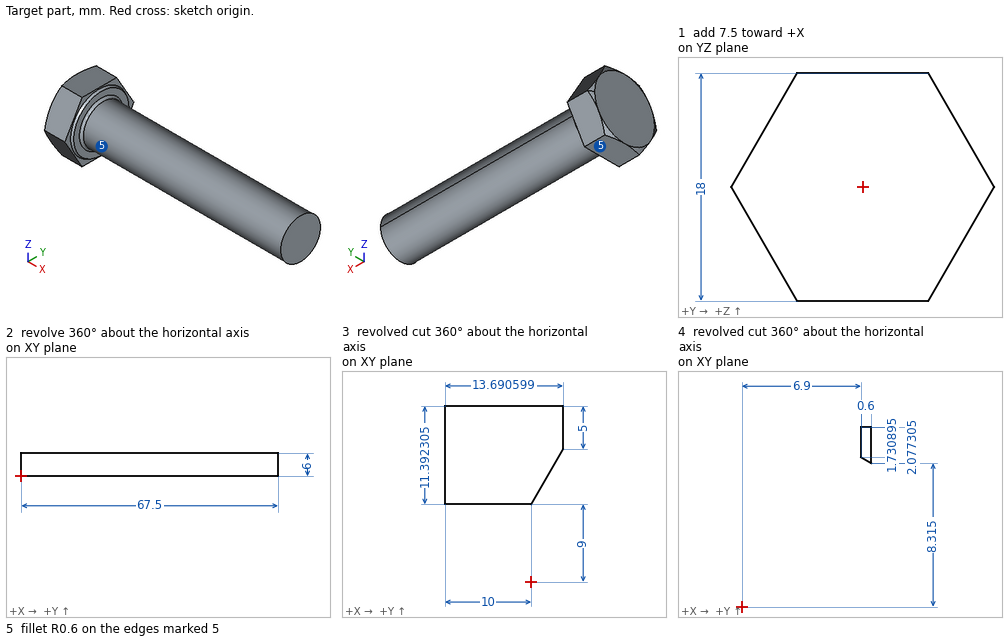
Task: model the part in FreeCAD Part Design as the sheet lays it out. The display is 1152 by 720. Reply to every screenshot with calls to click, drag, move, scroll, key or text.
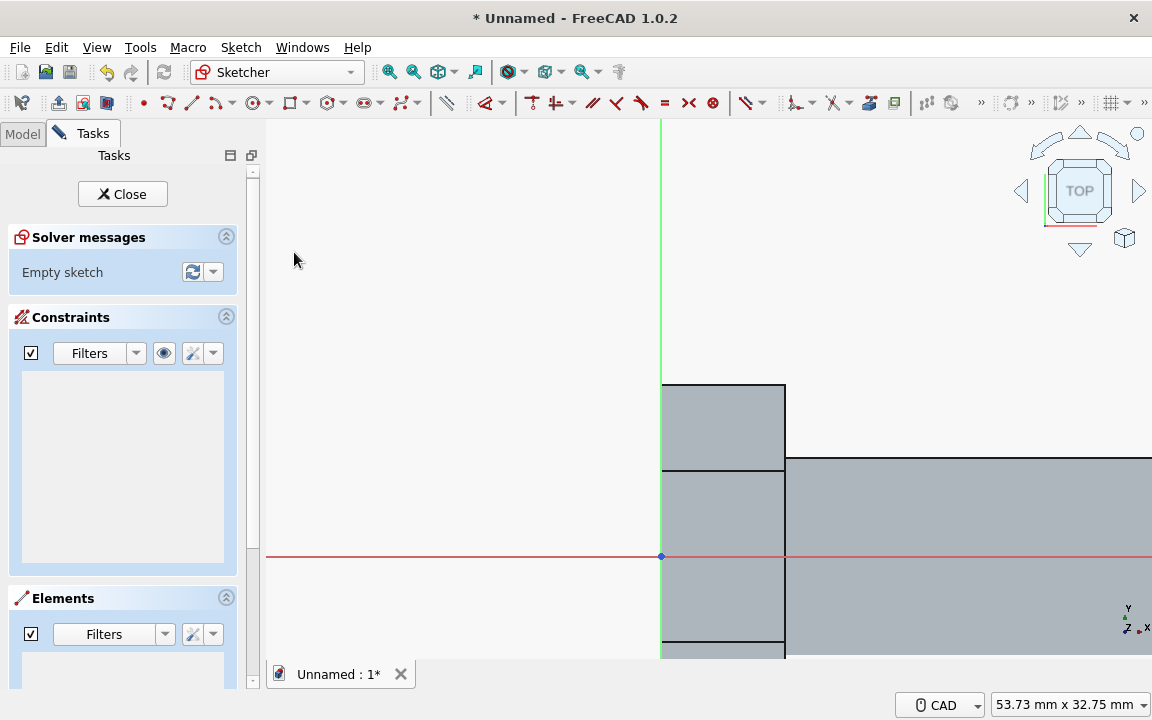
click(168, 104)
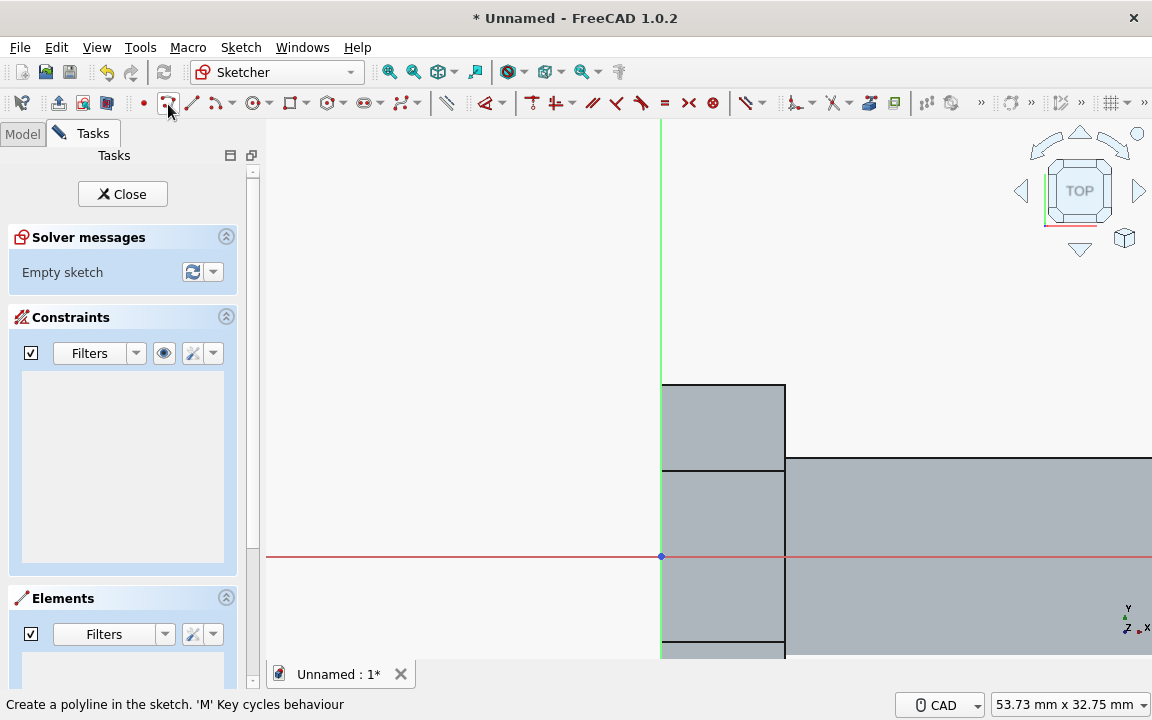
click(661, 408)
click(722, 303)
click(722, 220)
click(496, 220)
click(496, 408)
click(661, 409)
key(Escape)
key(Escape)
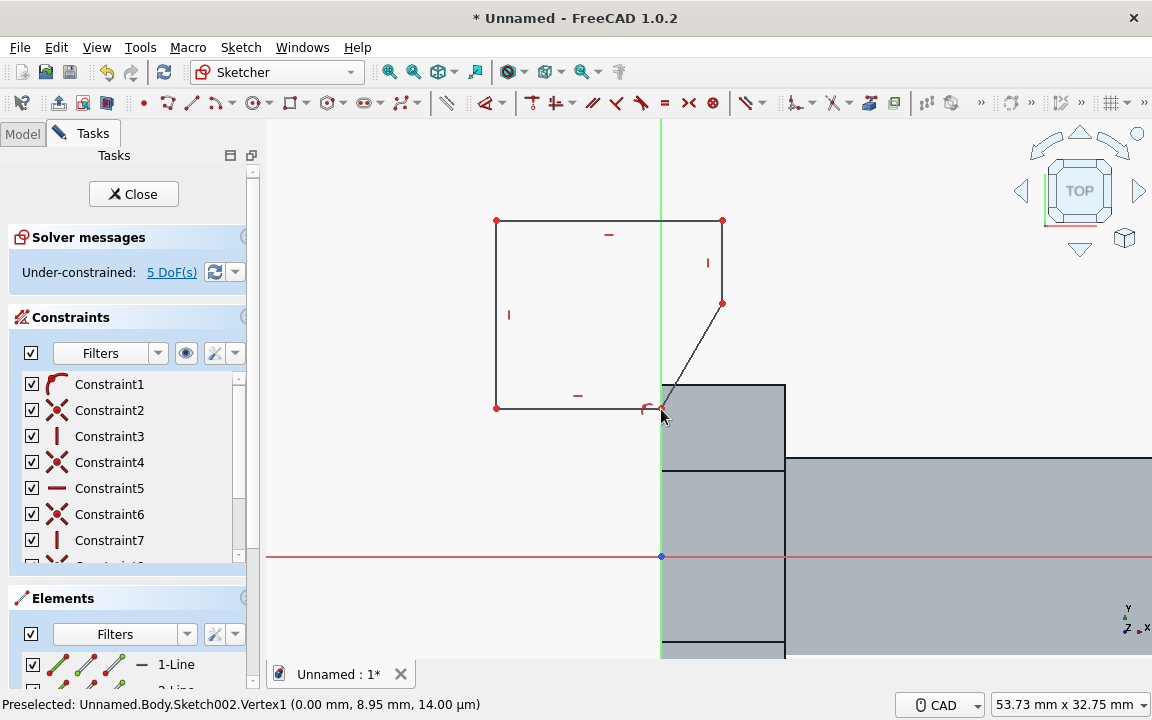
click(486, 104)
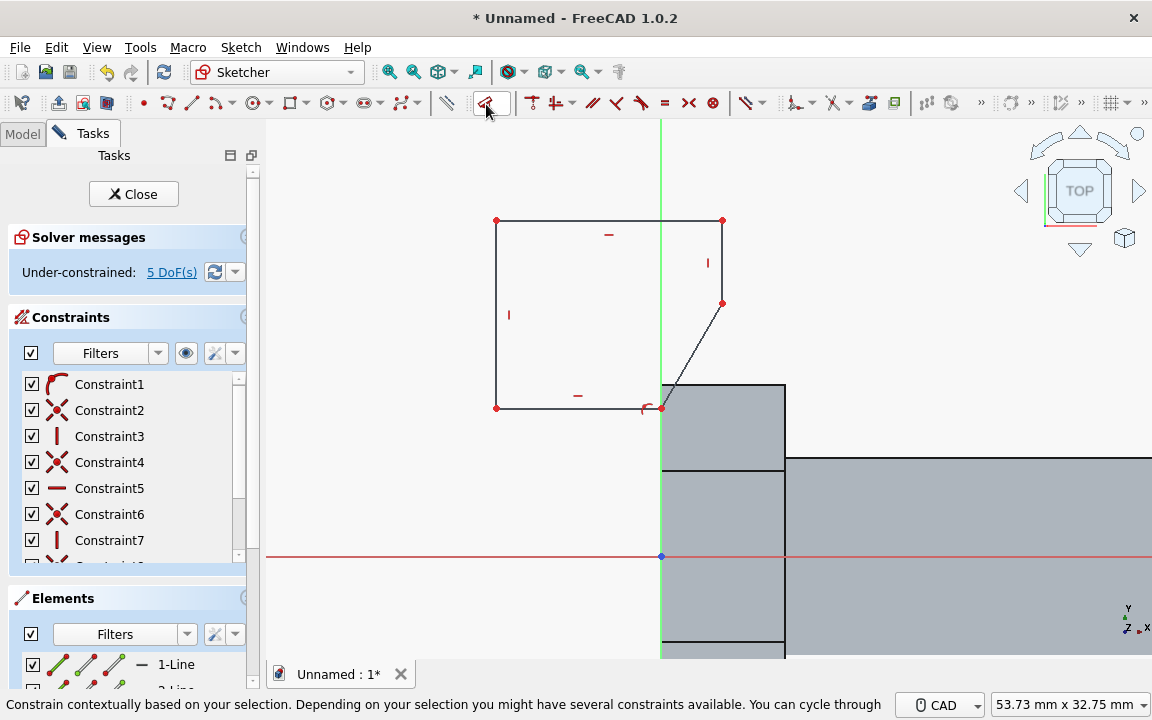
click(722, 279)
click(756, 262)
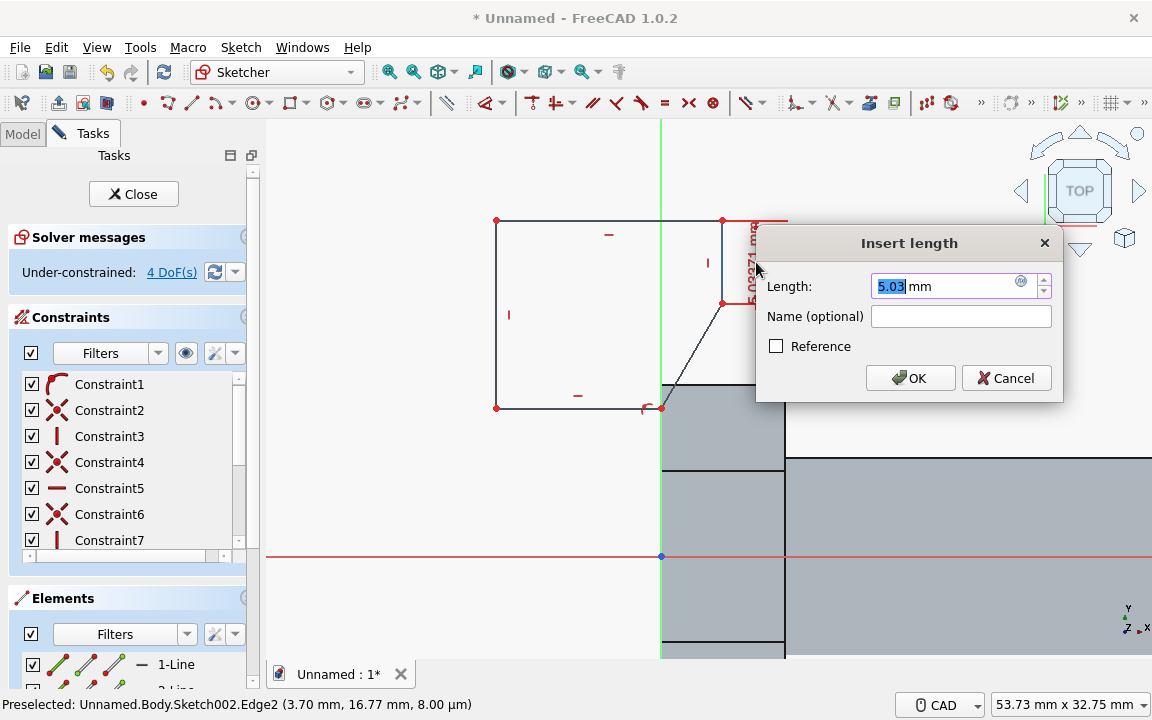
text(5)
key(Return)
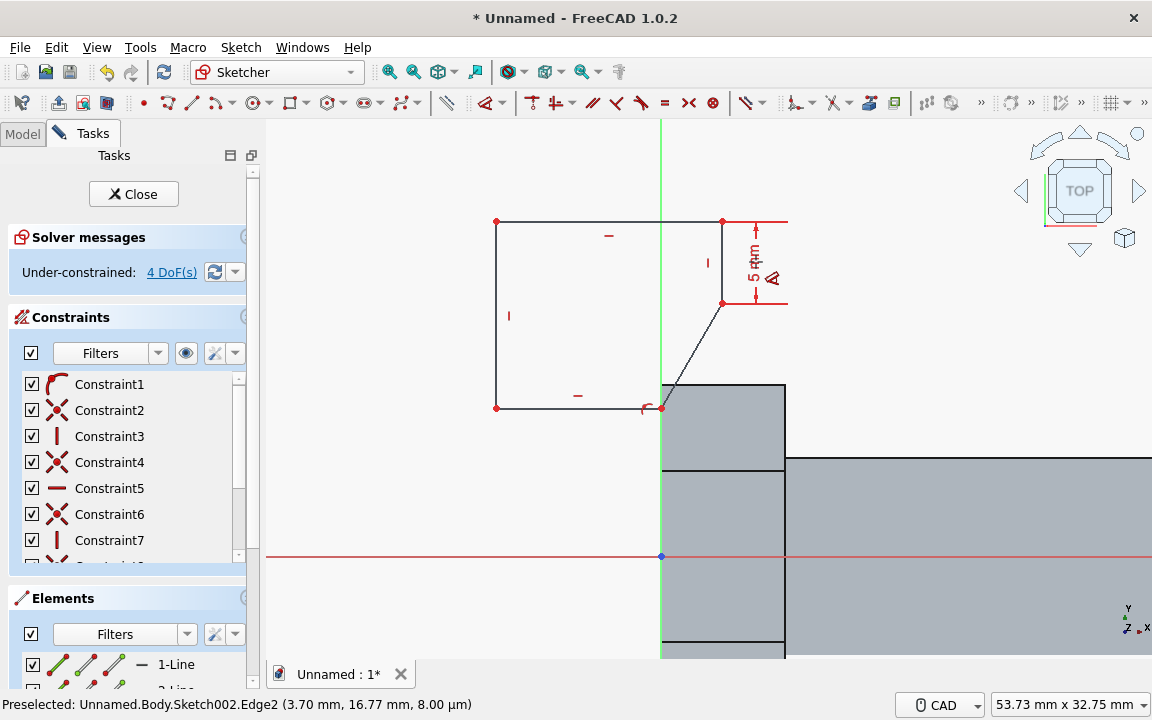
click(546, 409)
click(579, 443)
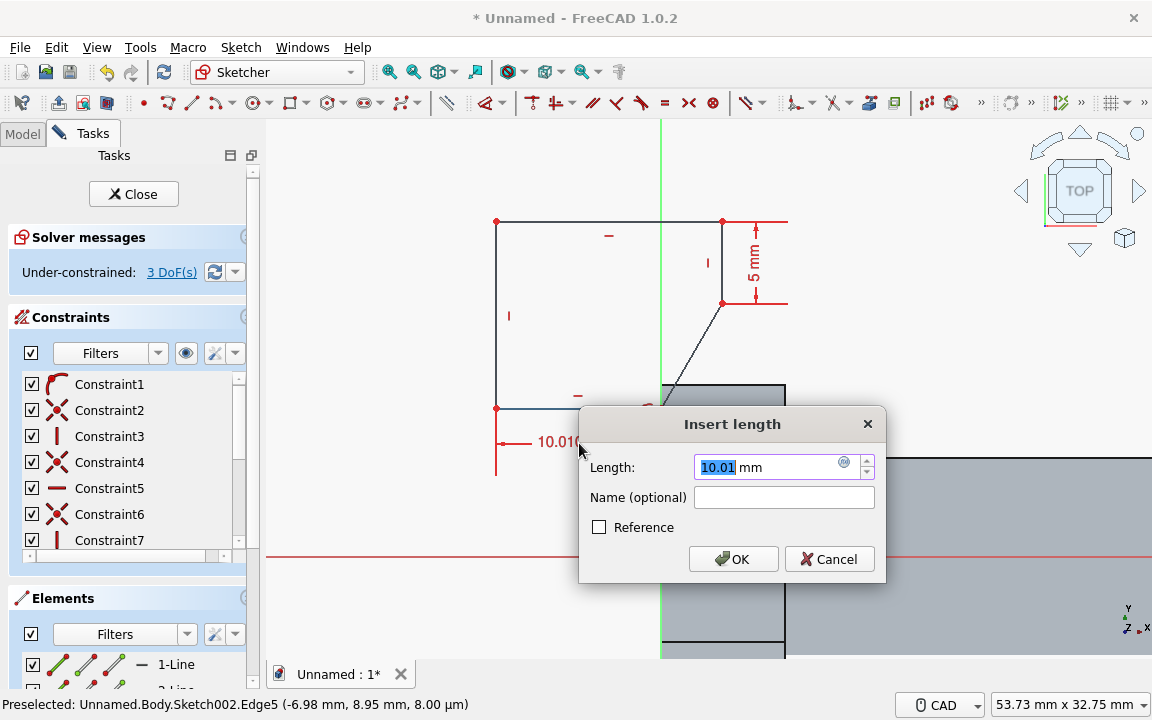
text(10)
key(Return)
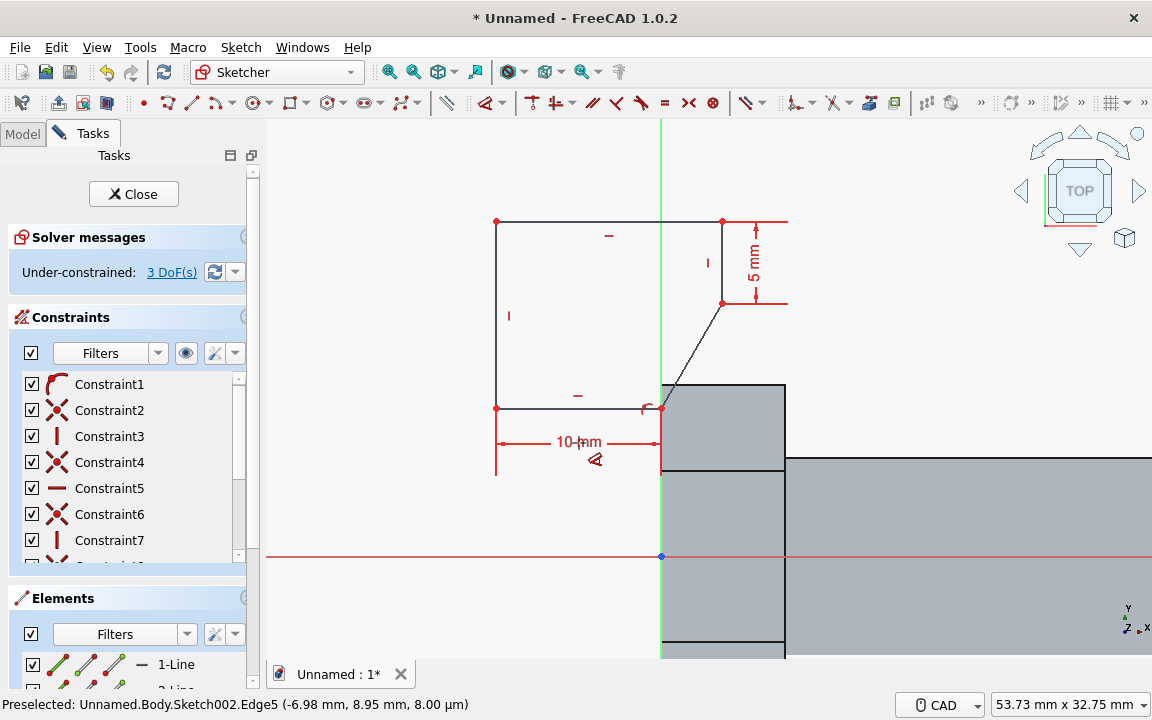
click(661, 409)
click(695, 483)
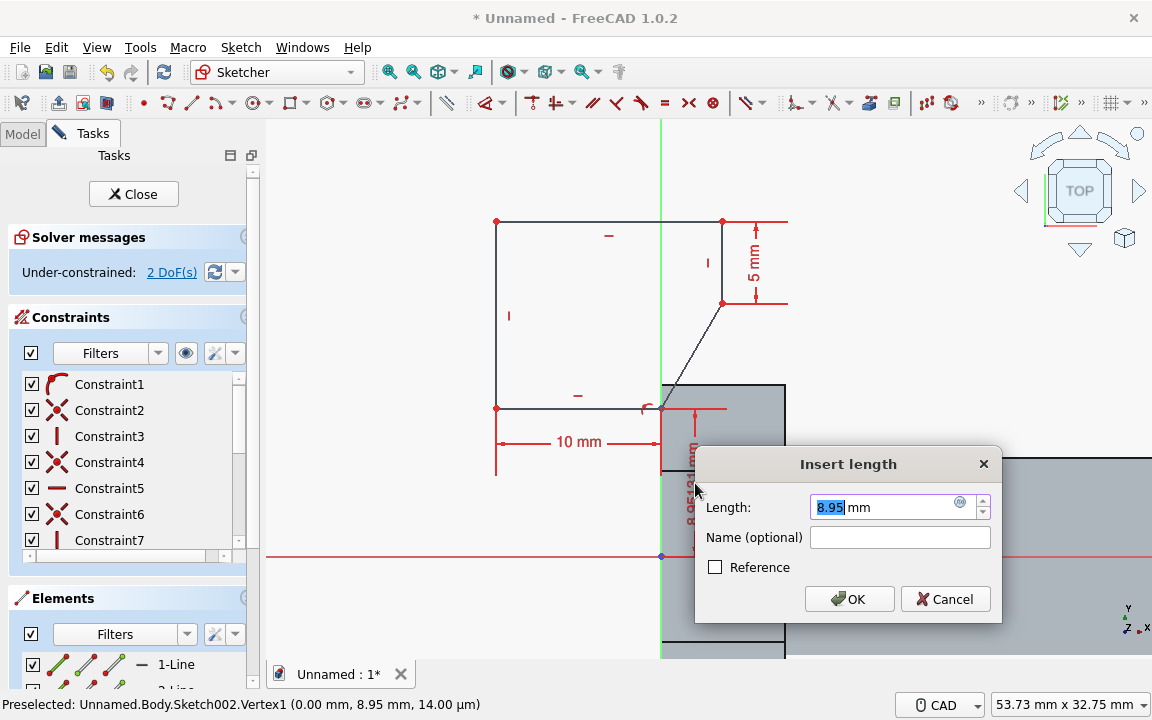
text(9)
key(Return)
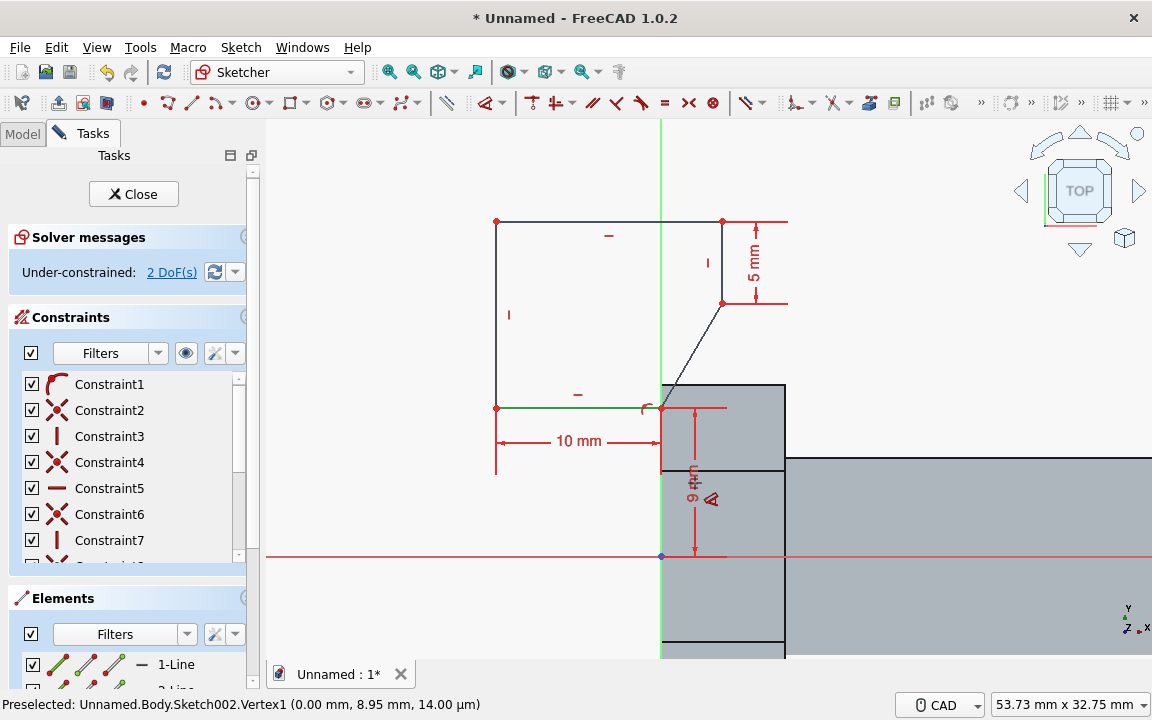
click(564, 222)
click(609, 188)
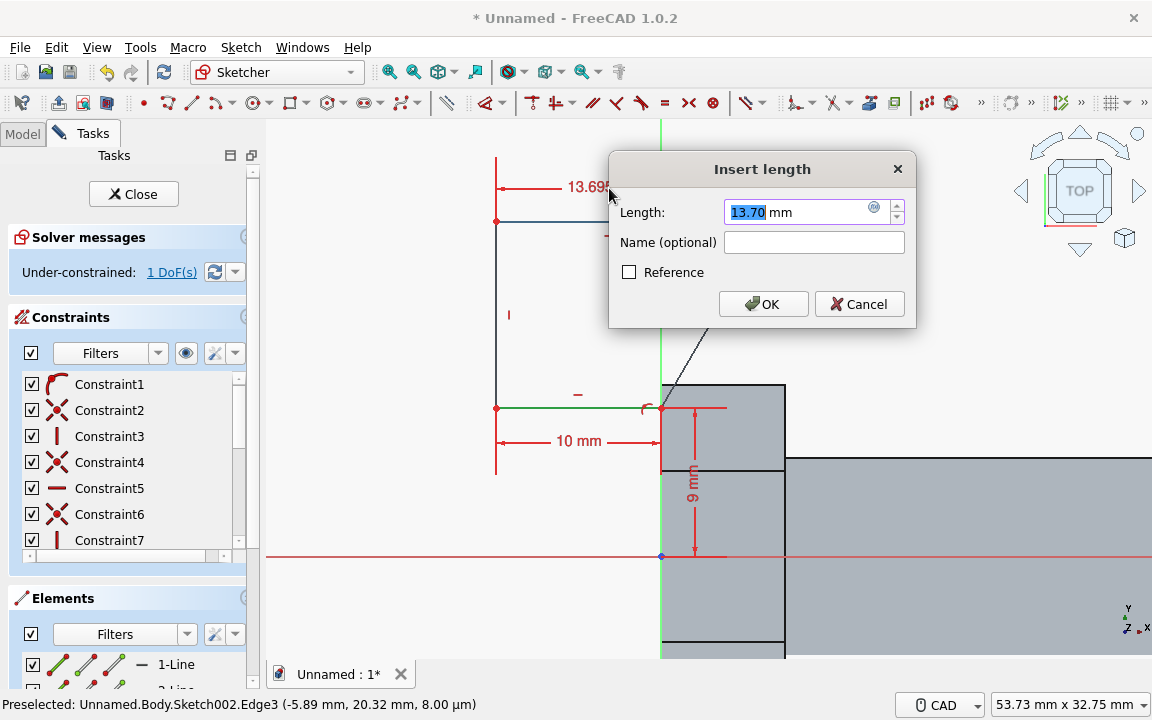
text(13.690599)
key(Return)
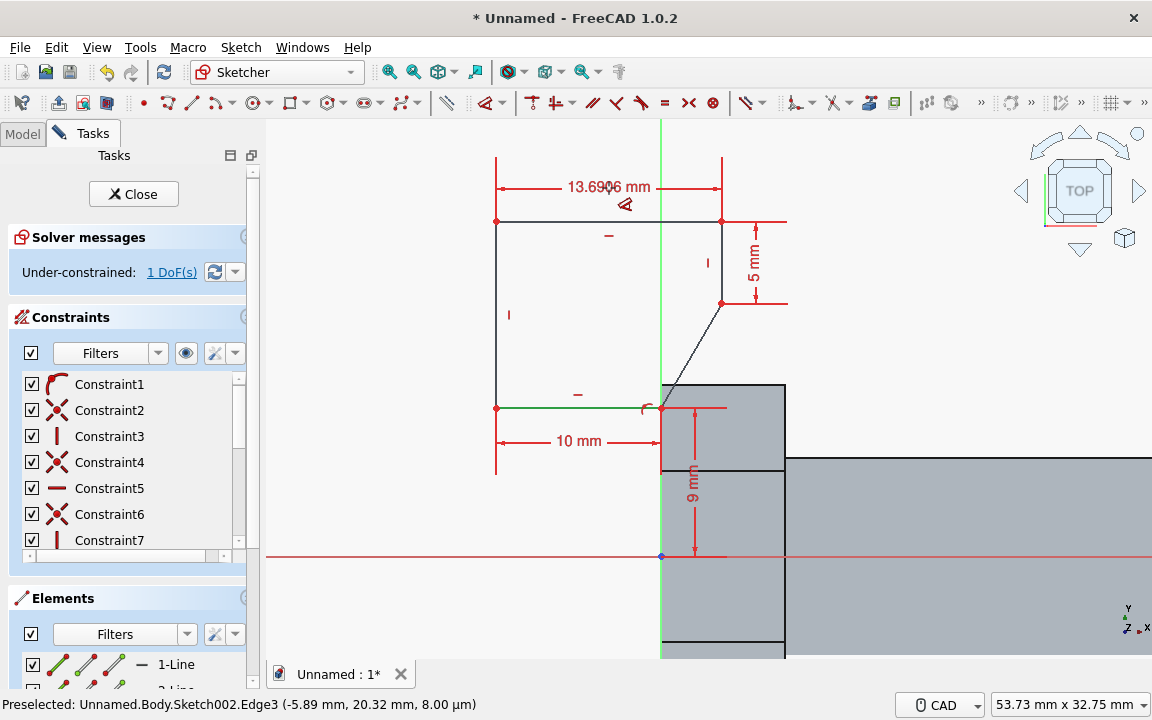
click(496, 278)
click(462, 315)